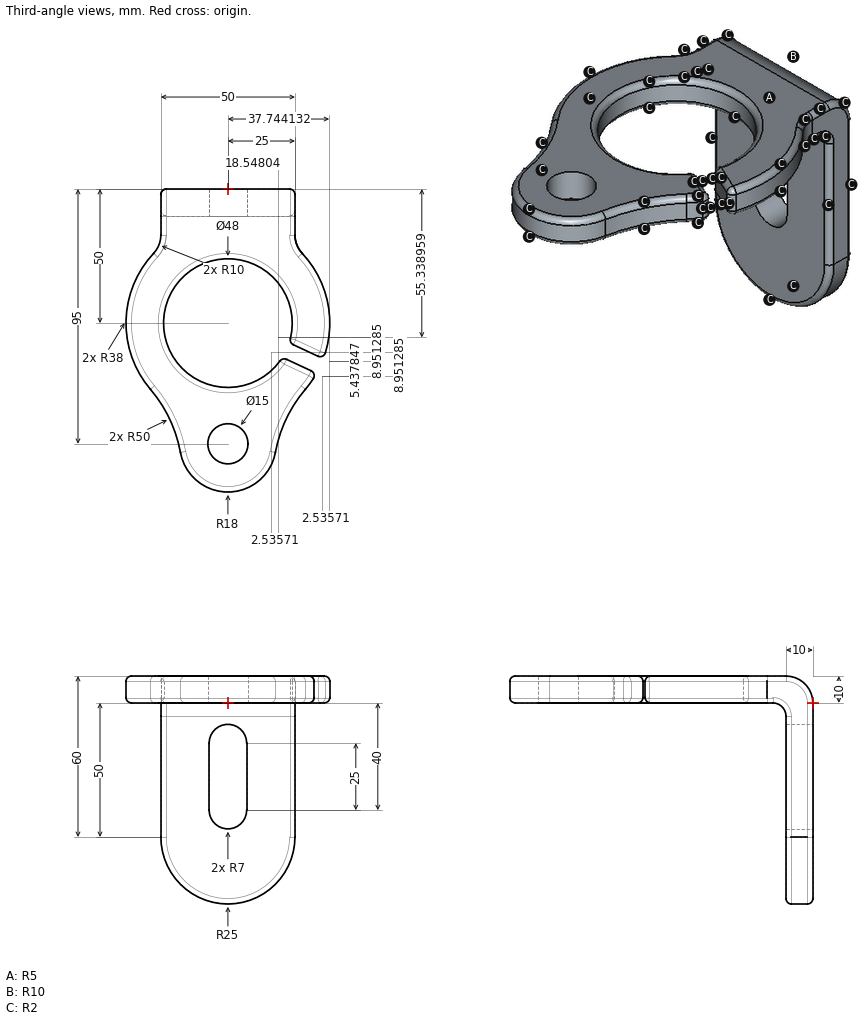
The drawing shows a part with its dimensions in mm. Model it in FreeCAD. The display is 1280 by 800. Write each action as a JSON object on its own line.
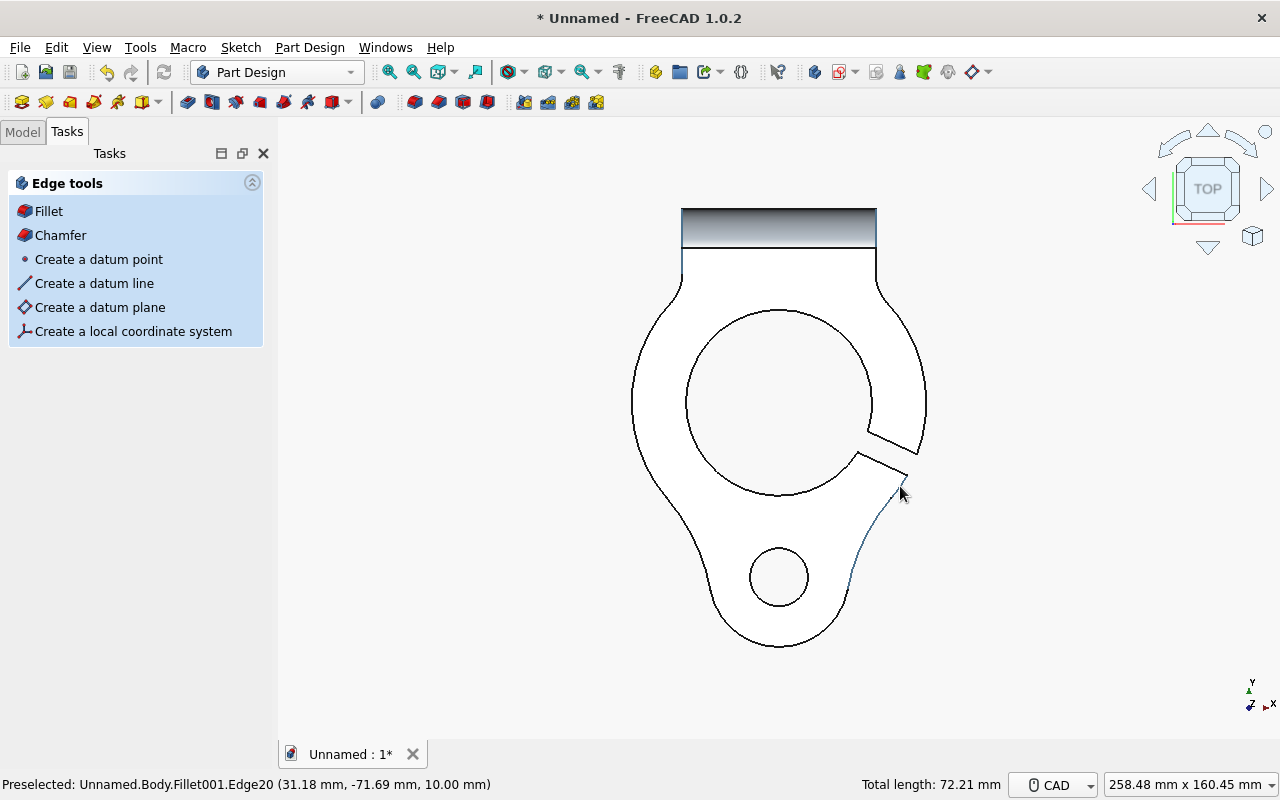
{"action": "left_click", "coordinate": [879, 289], "text": "ctrl"}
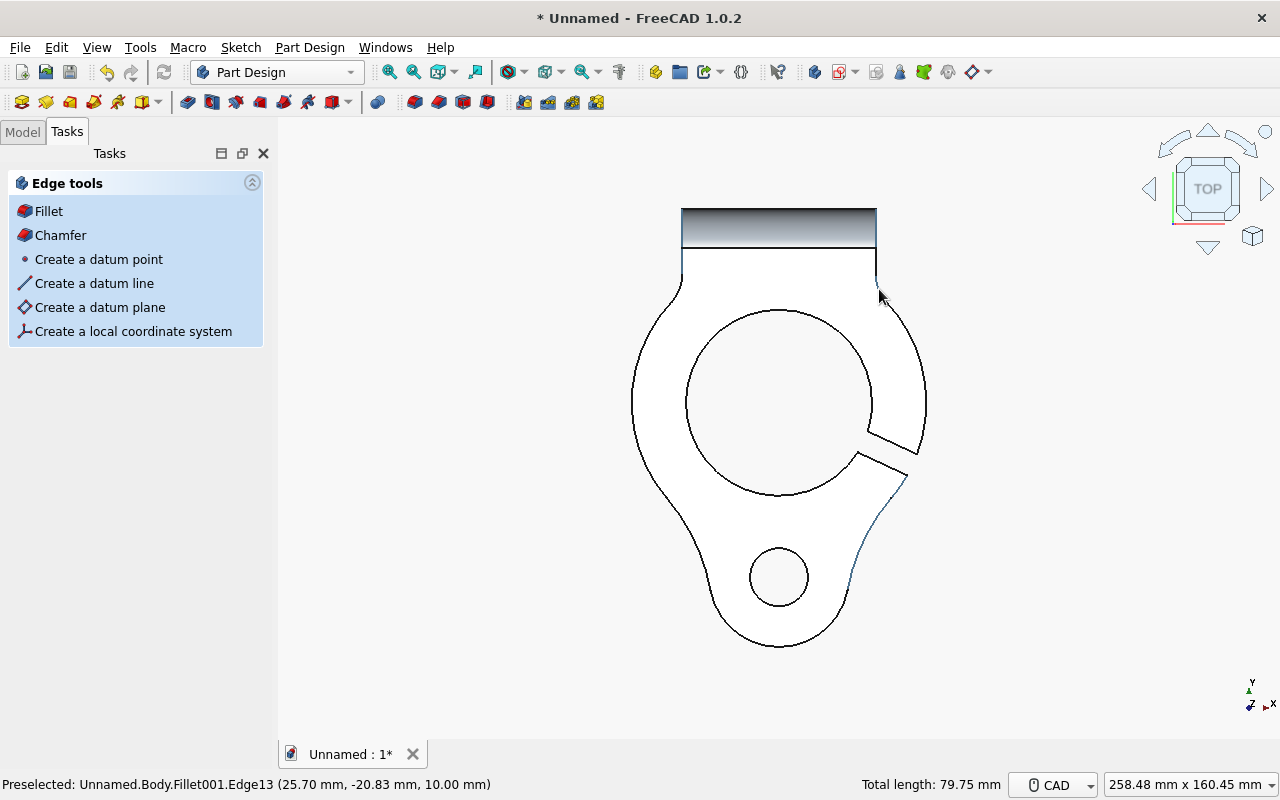
{"action": "left_click", "coordinate": [876, 261], "text": "ctrl"}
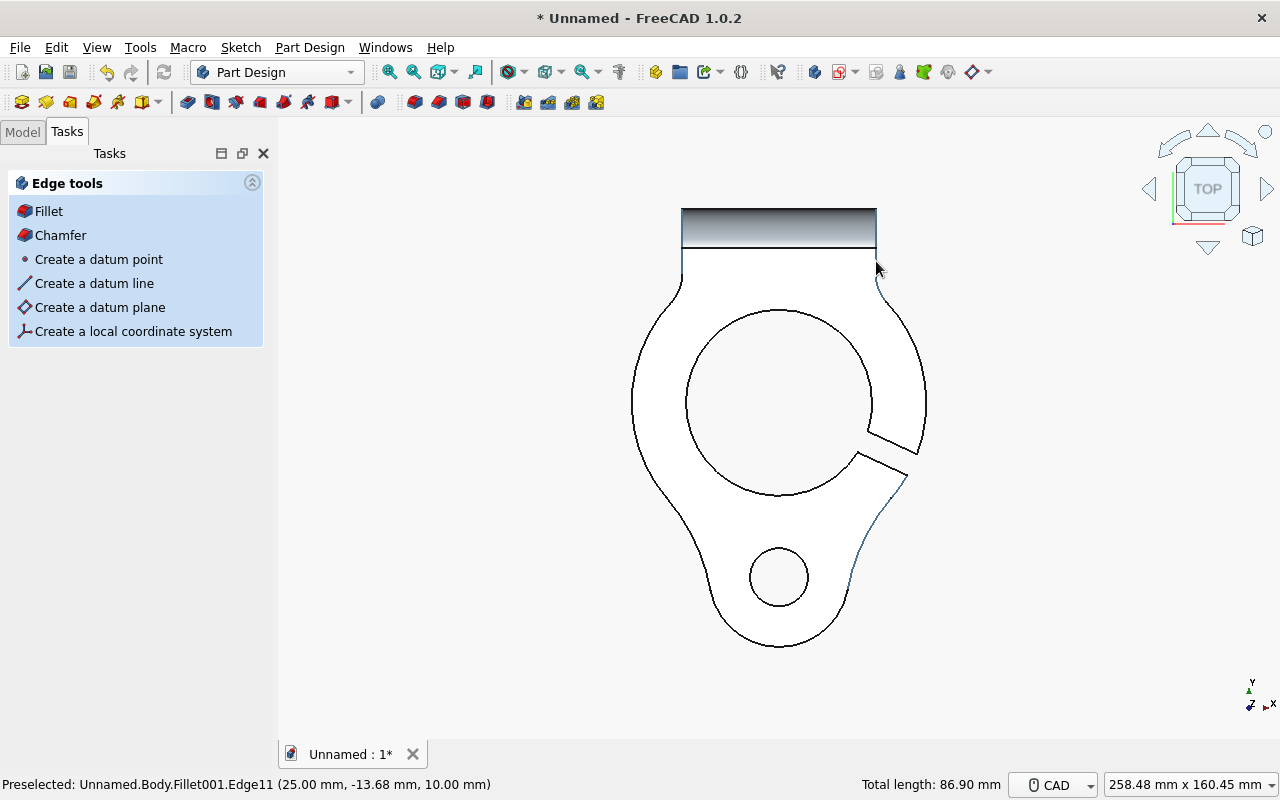
{"action": "left_click", "coordinate": [679, 289], "text": "ctrl"}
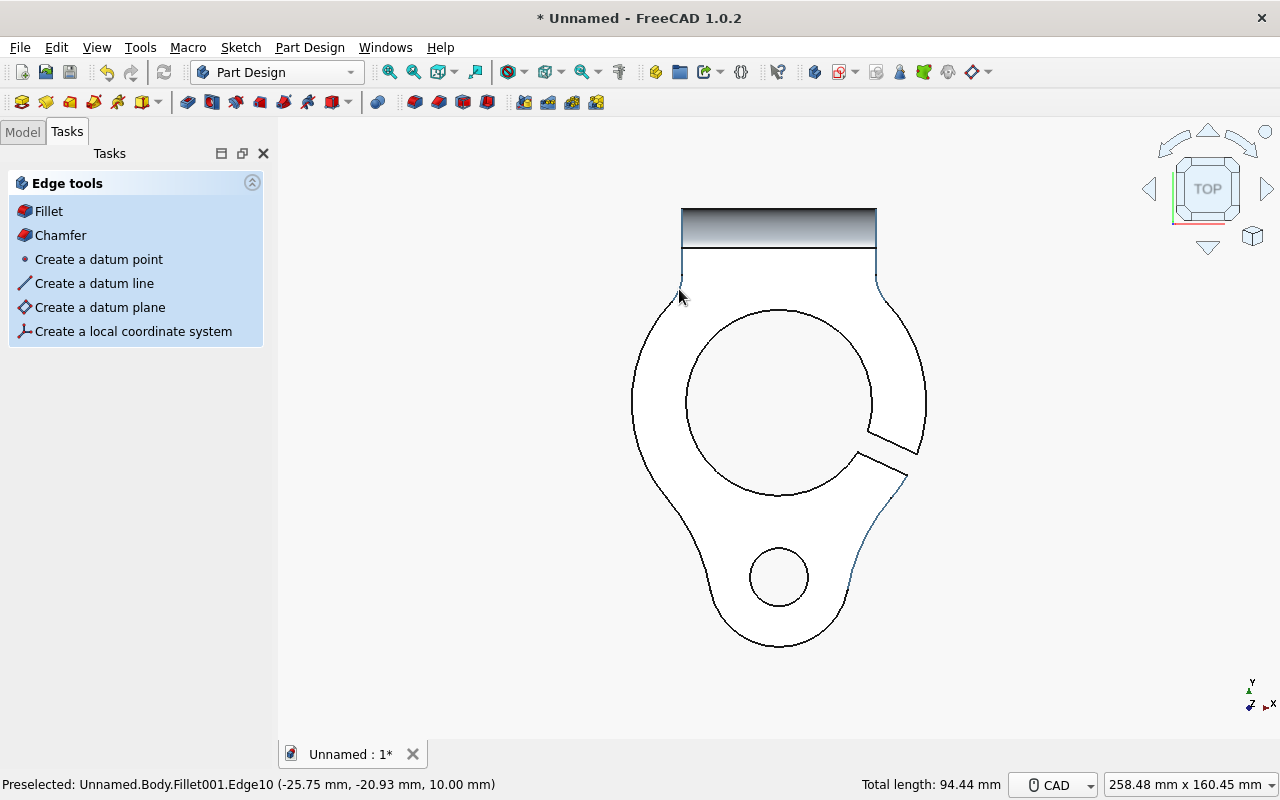
{"action": "left_click", "coordinate": [632, 398], "text": "ctrl"}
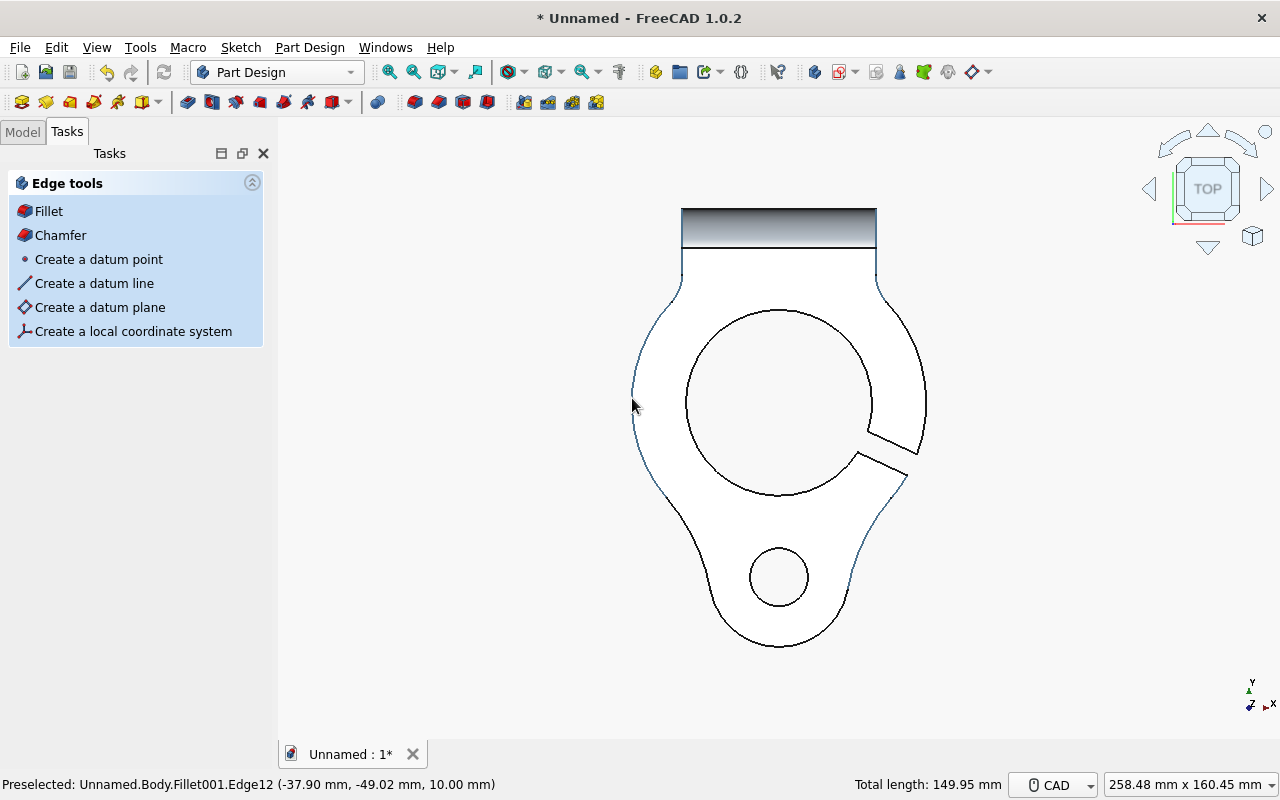
{"action": "left_click", "coordinate": [695, 540], "text": "ctrl"}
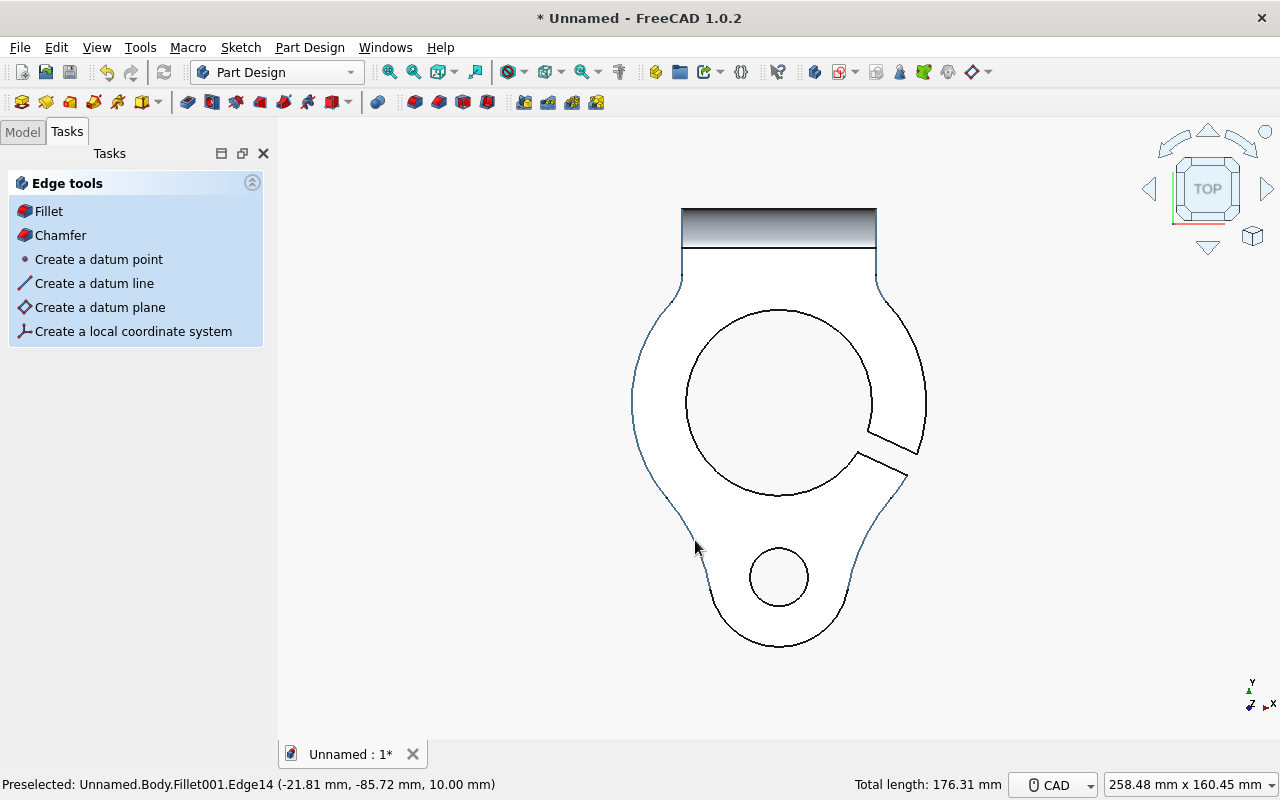
{"action": "left_click", "coordinate": [690, 376], "text": "ctrl"}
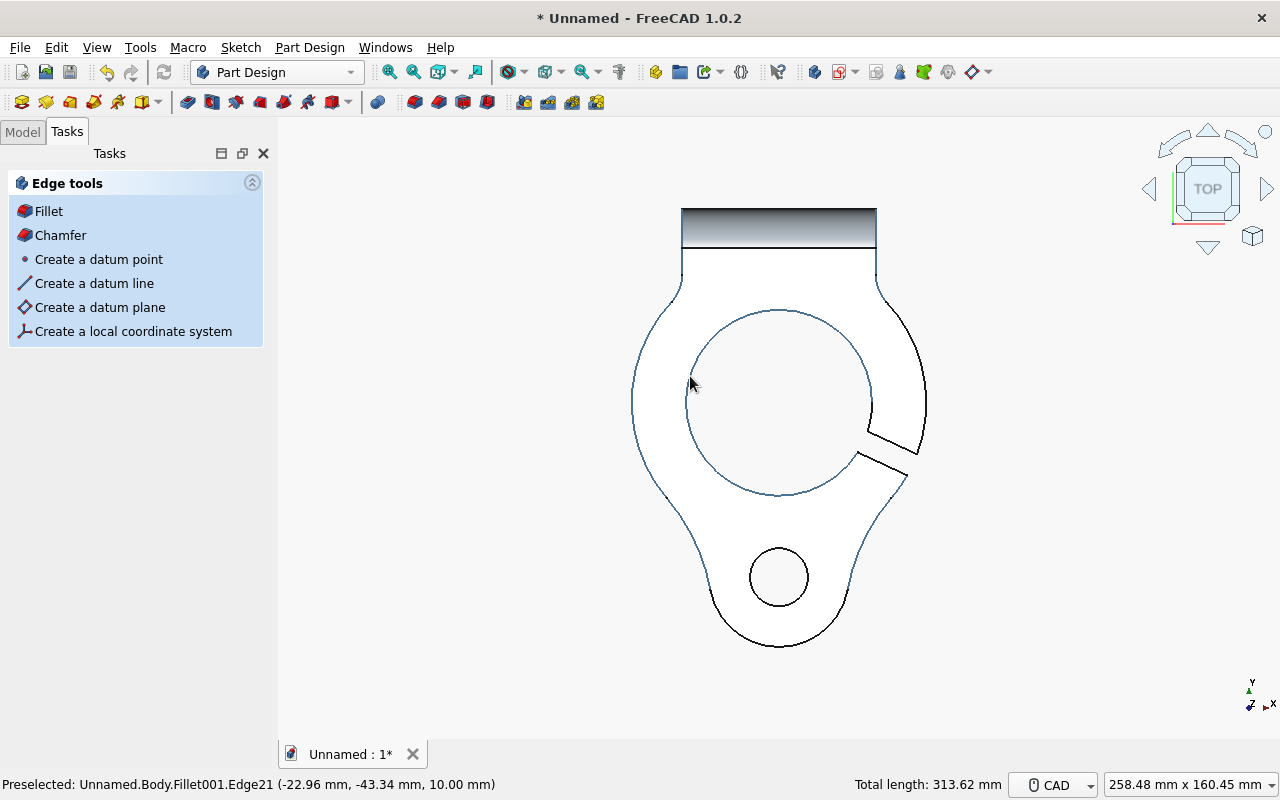
{"action": "left_click", "coordinate": [923, 373], "text": "ctrl"}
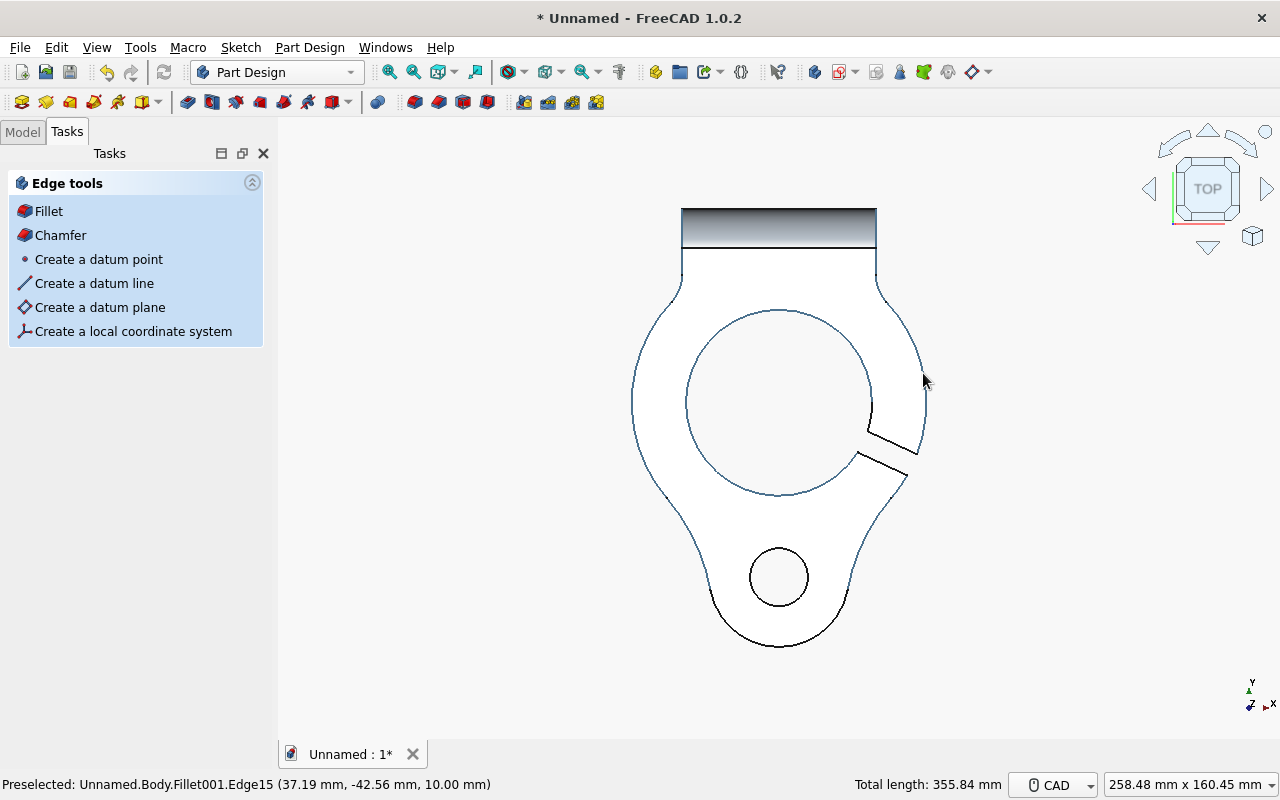
{"action": "left_click", "coordinate": [779, 646], "text": "ctrl"}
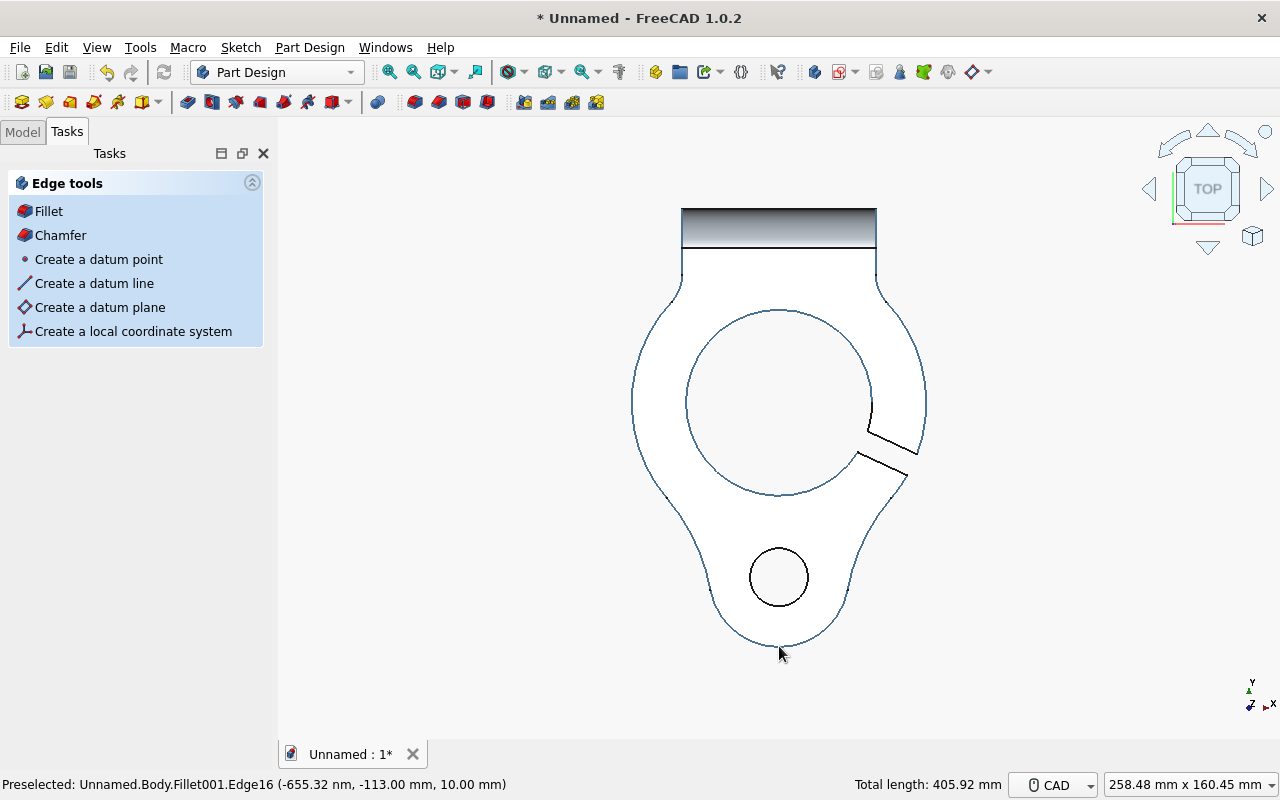
{"action": "key", "text": "0"}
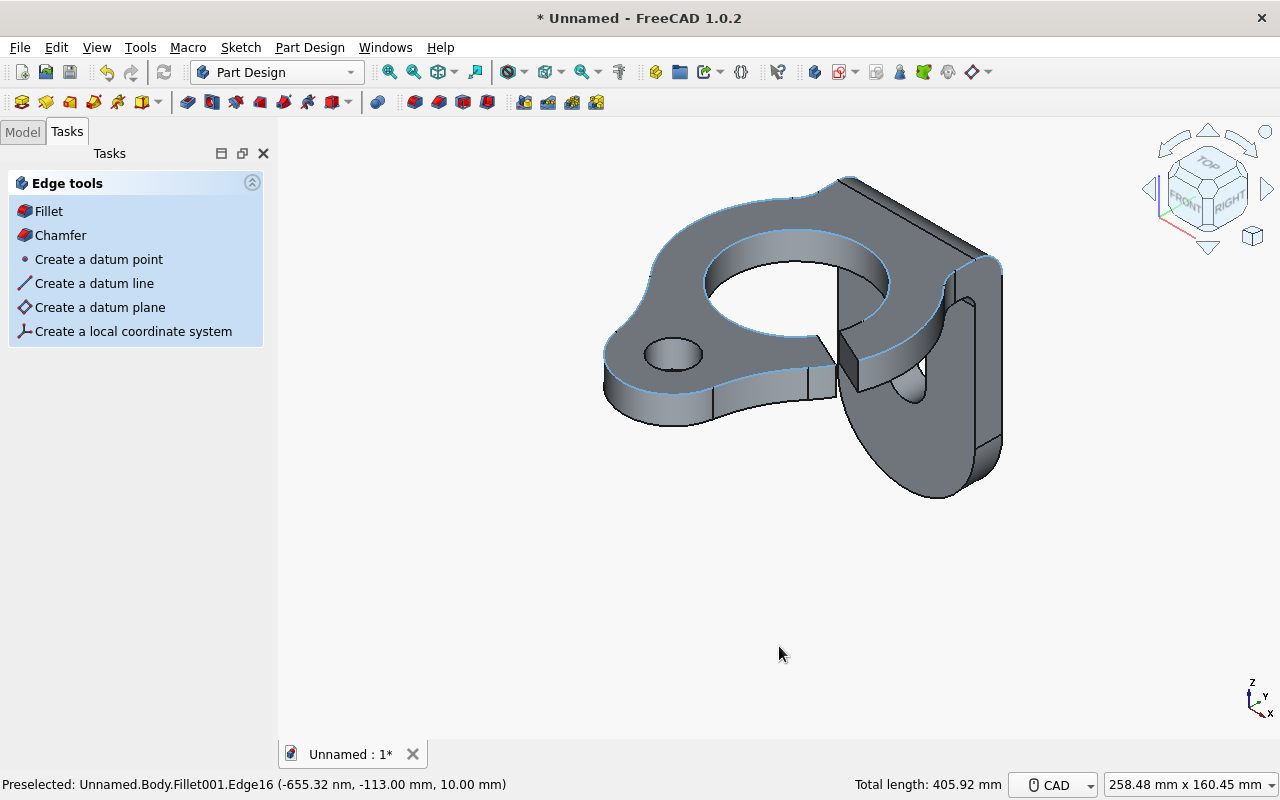
{"action": "left_click", "coordinate": [849, 365], "text": "ctrl"}